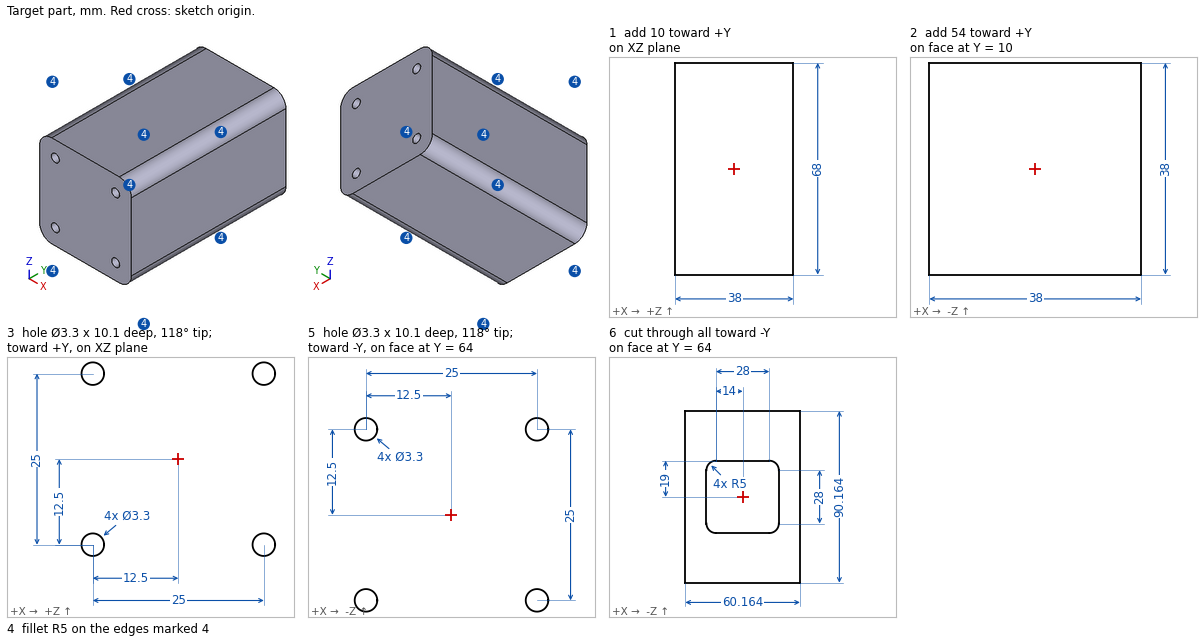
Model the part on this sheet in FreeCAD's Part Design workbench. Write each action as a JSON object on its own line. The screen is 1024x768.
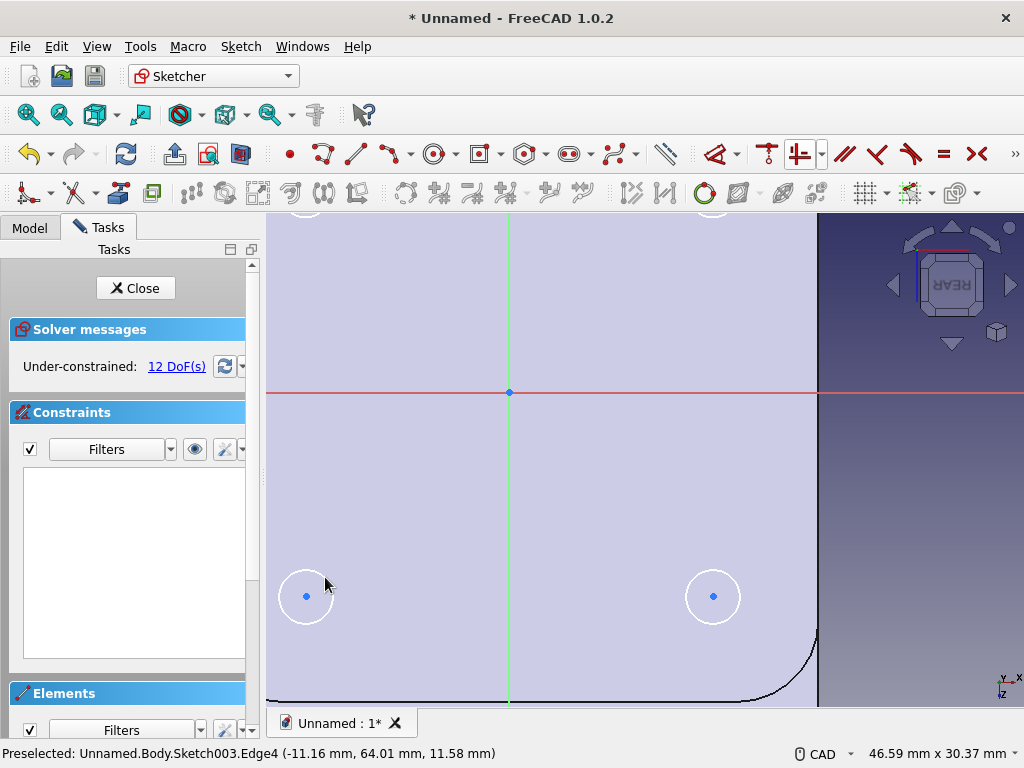
{"action": "scroll", "coordinate": [713, 597], "scroll_direction": "down", "scroll_amount": 2}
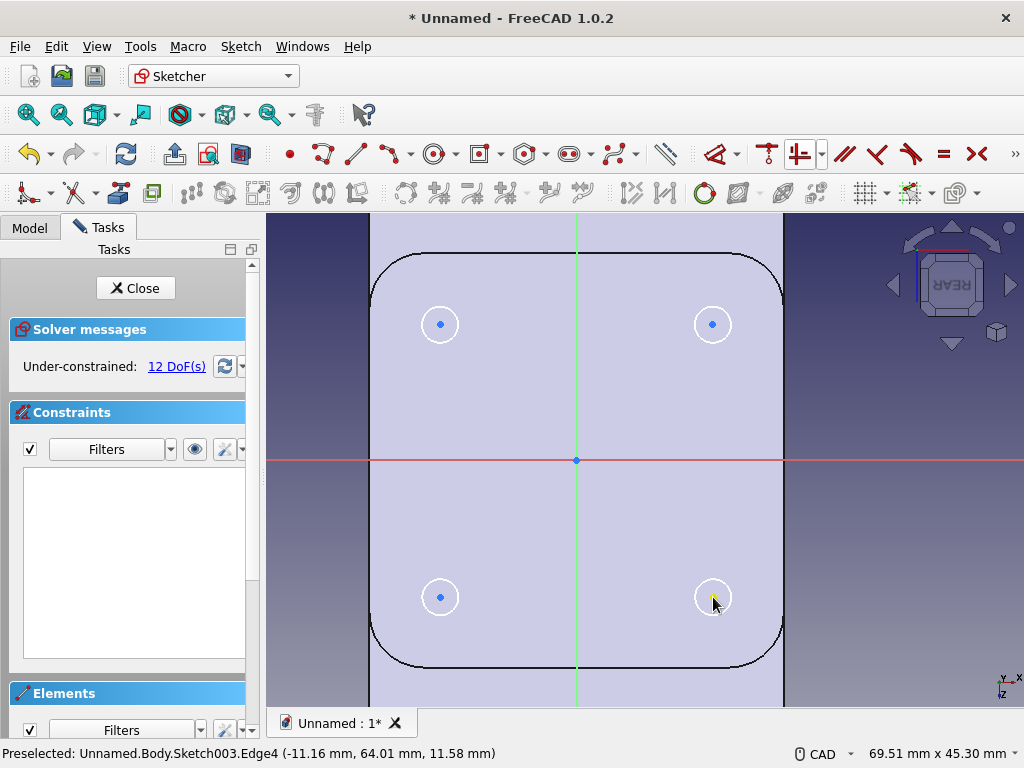
{"action": "left_click", "coordinate": [453, 312]}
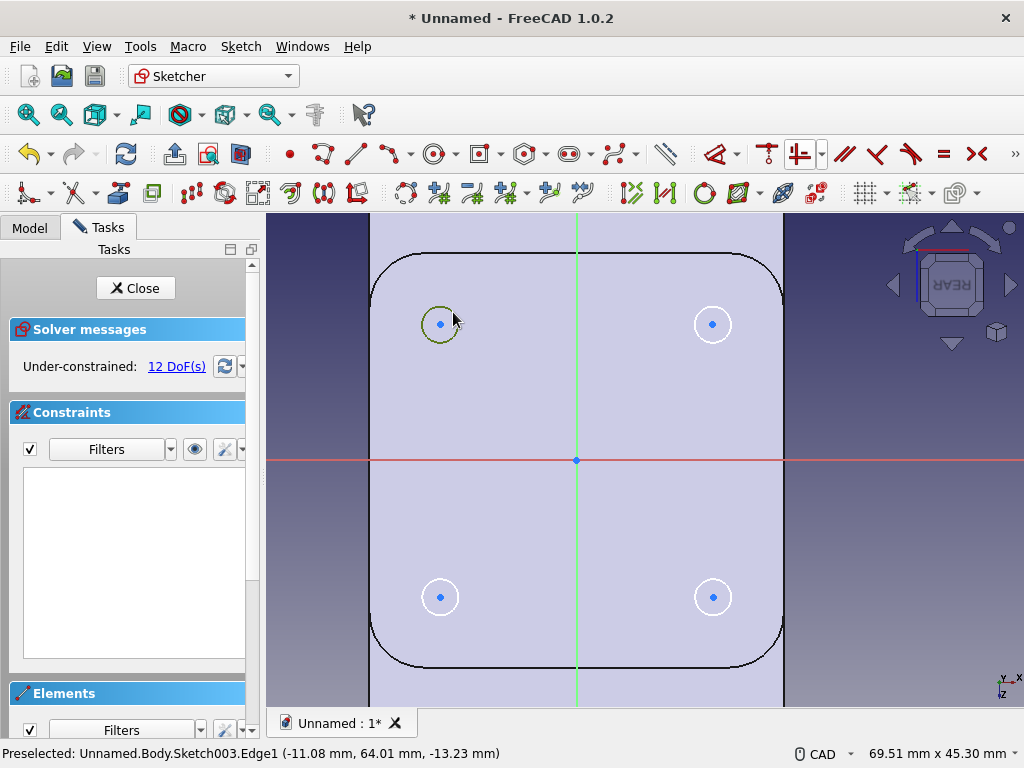
{"action": "left_click", "coordinate": [726, 312]}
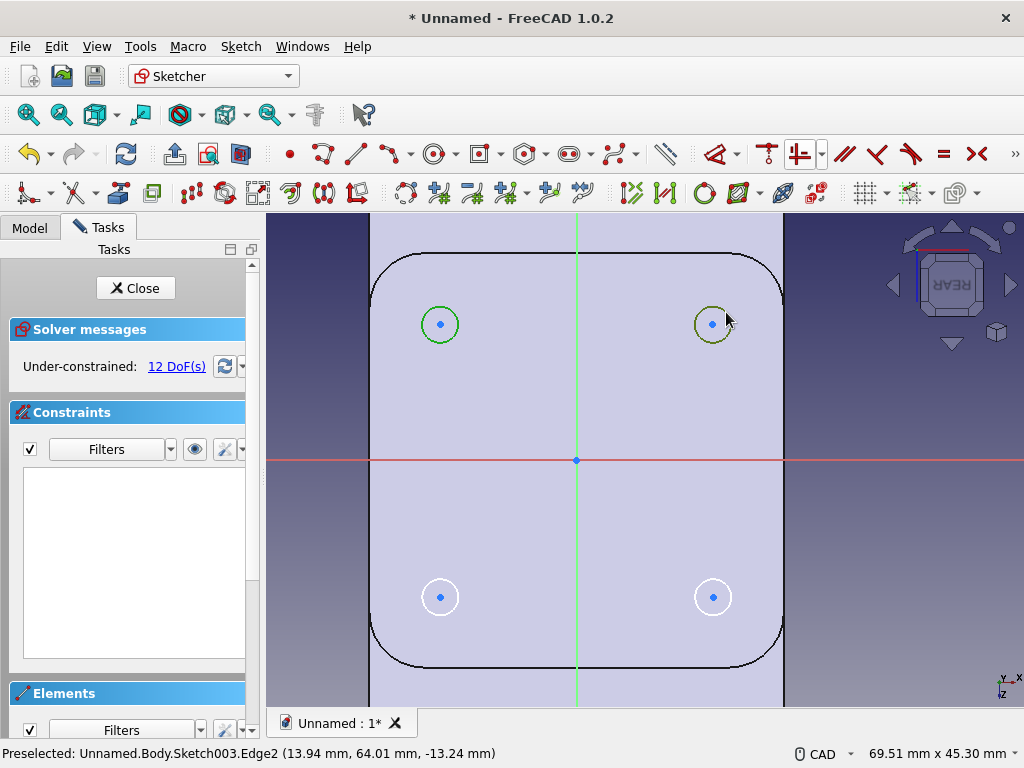
{"action": "left_click", "coordinate": [726, 584]}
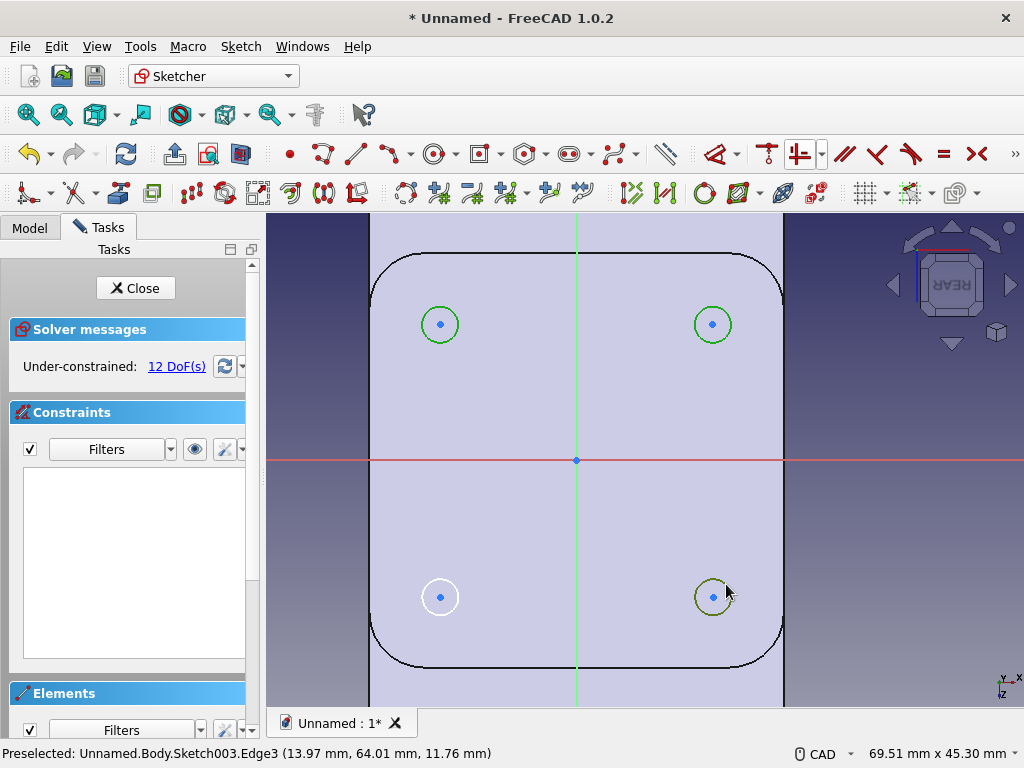
{"action": "left_click", "coordinate": [453, 584]}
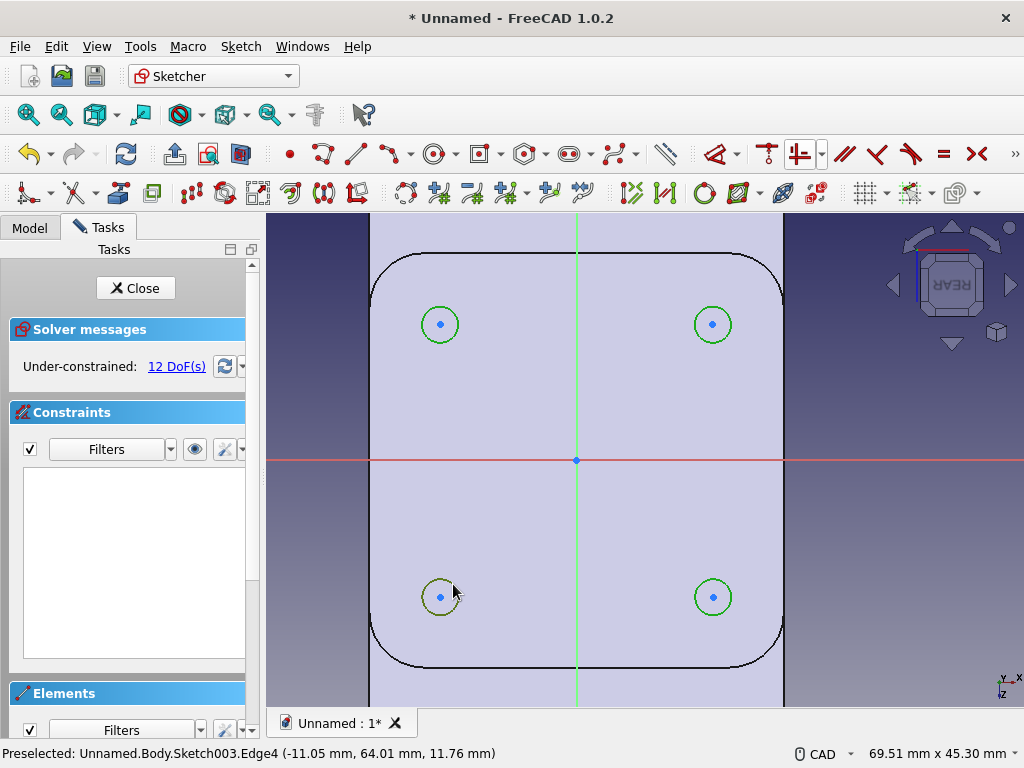
{"action": "left_click", "coordinate": [944, 154]}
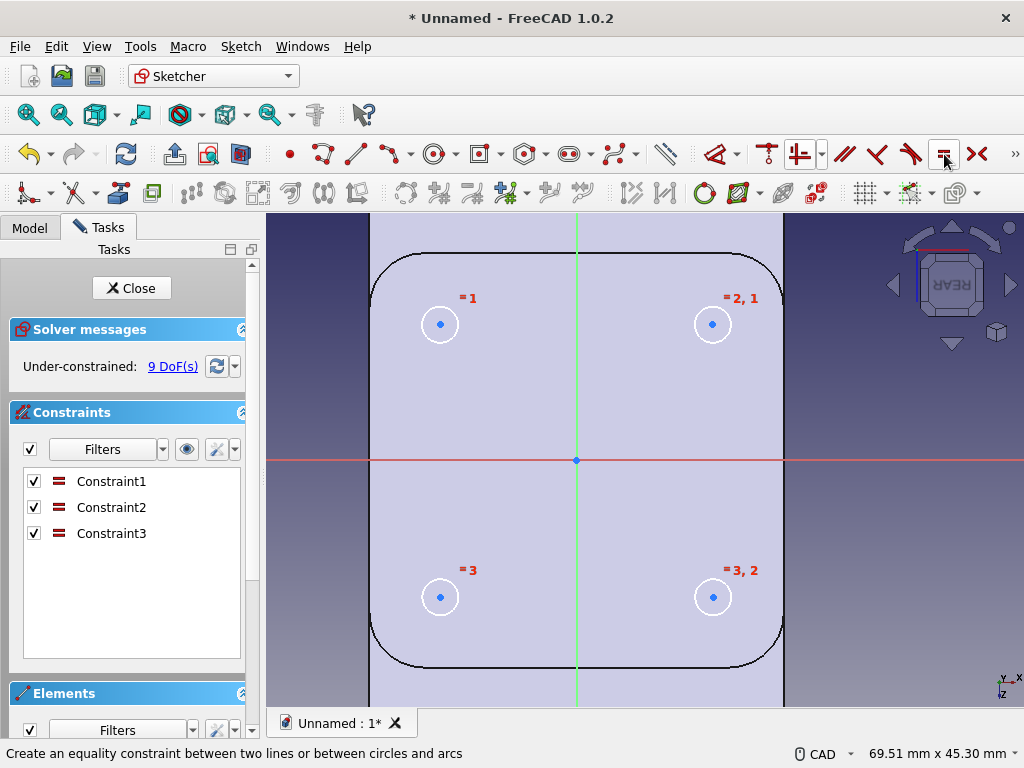
{"action": "left_click", "coordinate": [440, 325]}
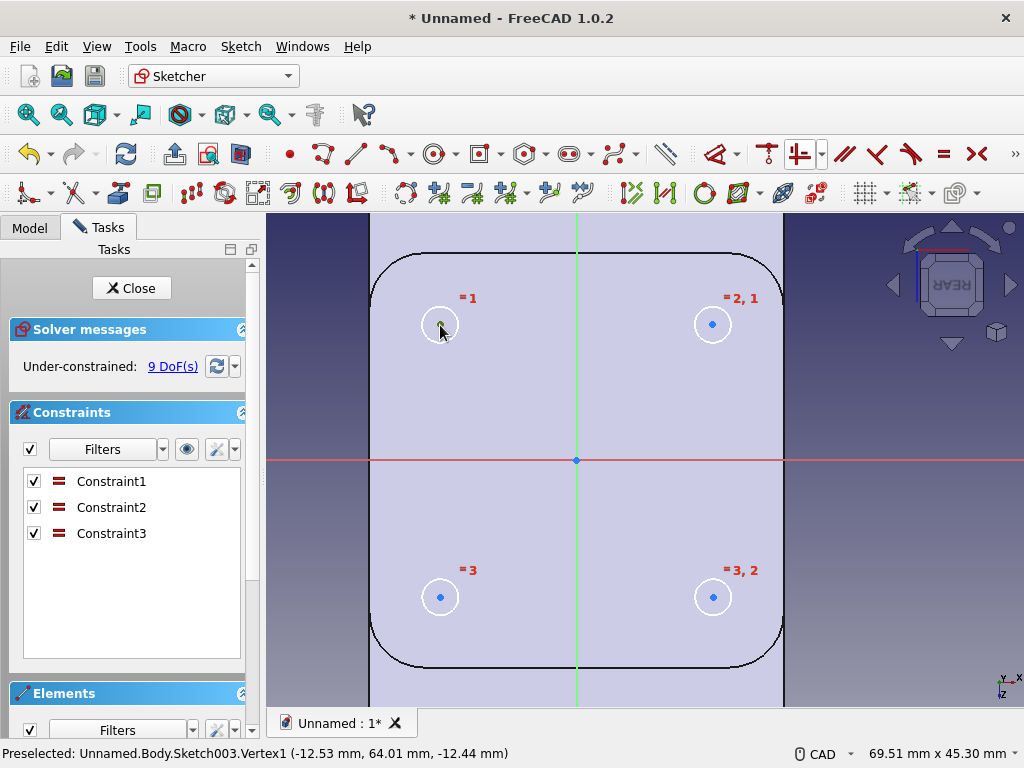
{"action": "left_click", "coordinate": [713, 325]}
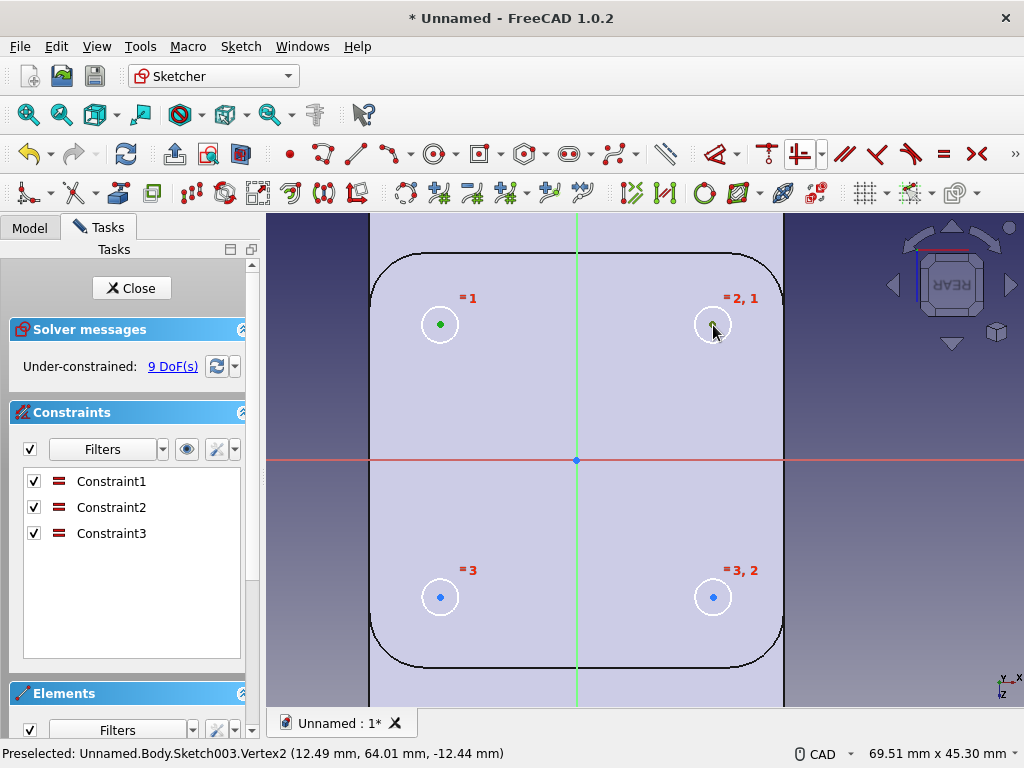
{"action": "key", "text": "h"}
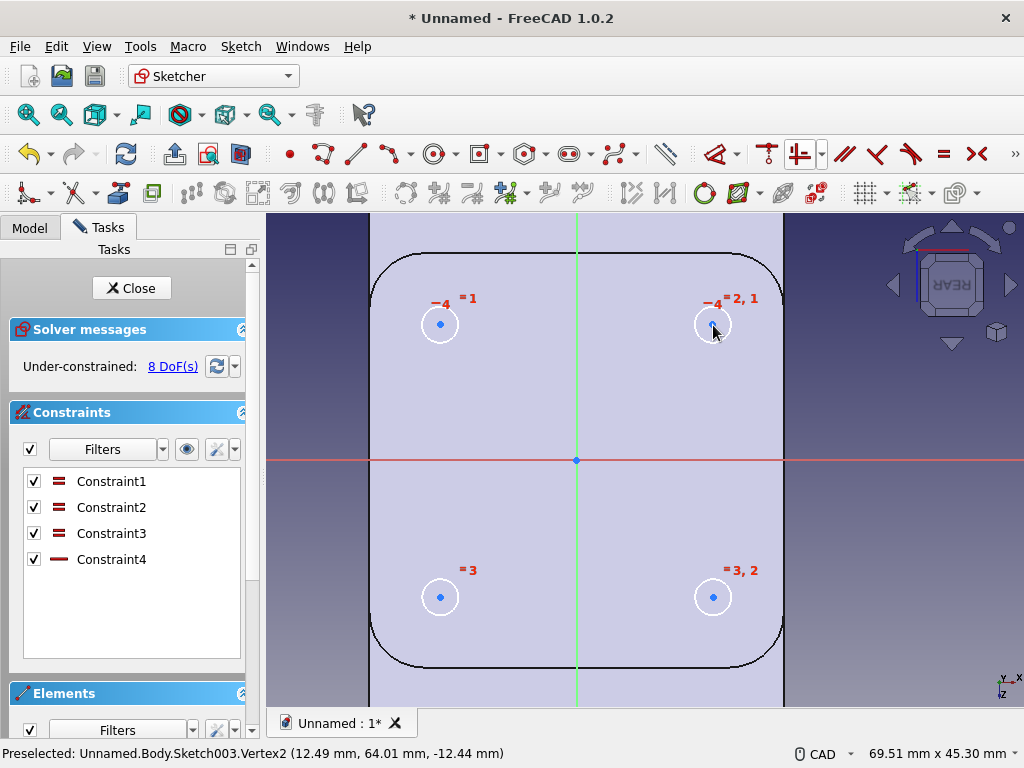
{"action": "left_click", "coordinate": [713, 325]}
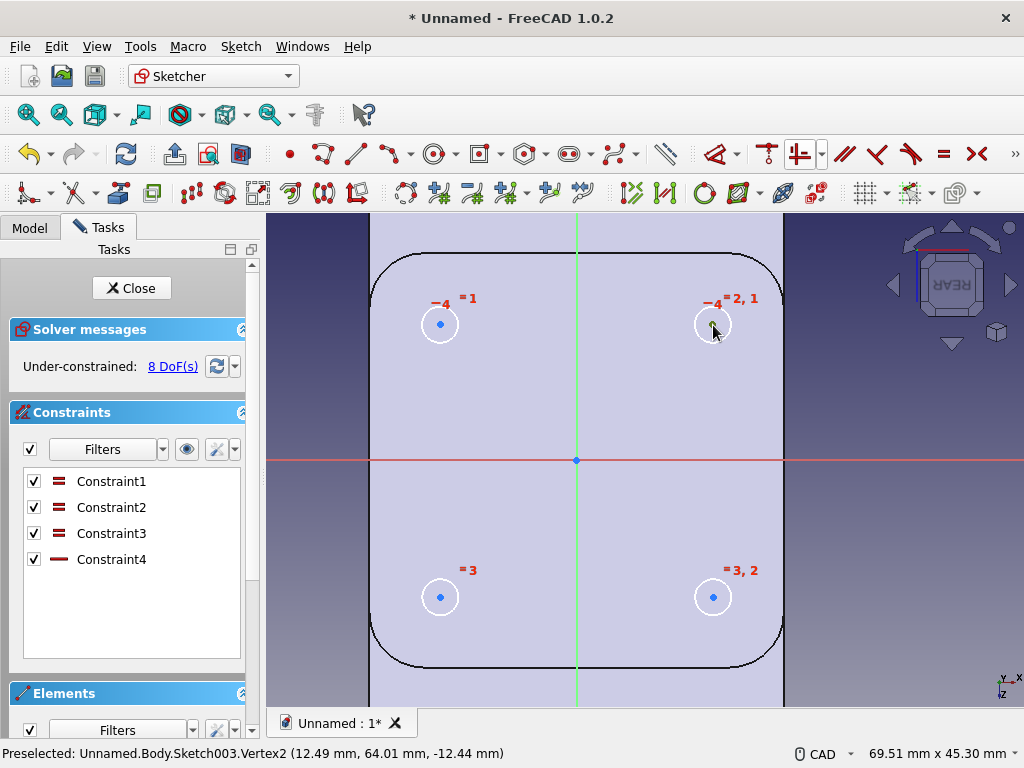
{"action": "left_click", "coordinate": [713, 597]}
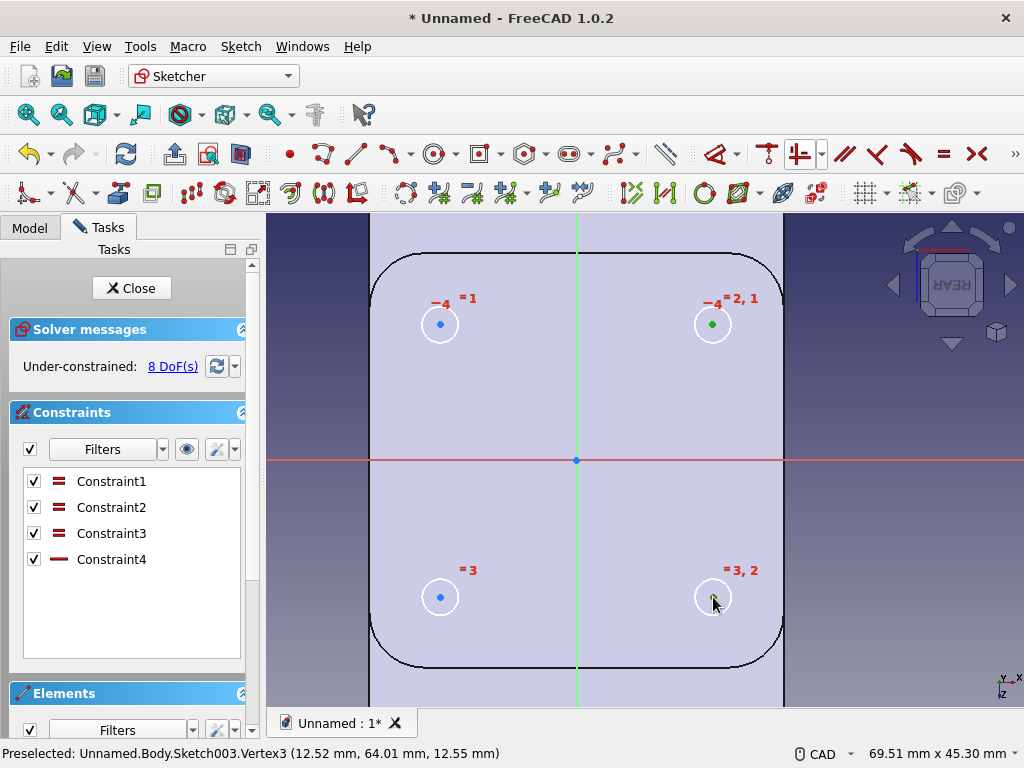
{"action": "key", "text": "v"}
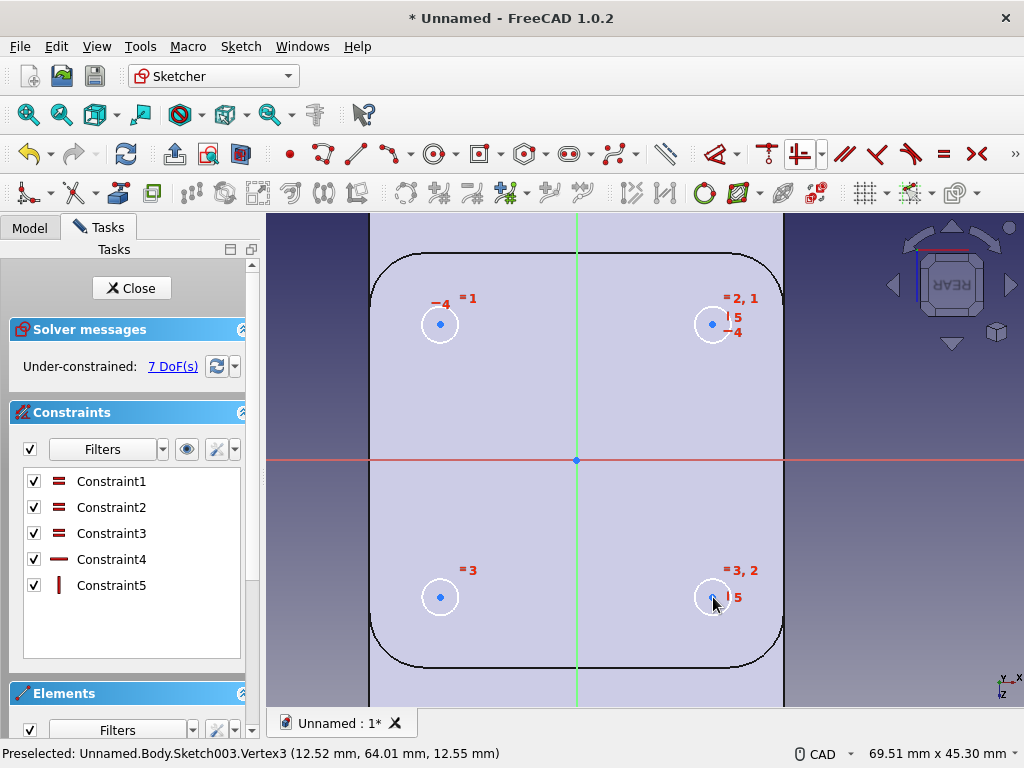
{"action": "left_click", "coordinate": [440, 325]}